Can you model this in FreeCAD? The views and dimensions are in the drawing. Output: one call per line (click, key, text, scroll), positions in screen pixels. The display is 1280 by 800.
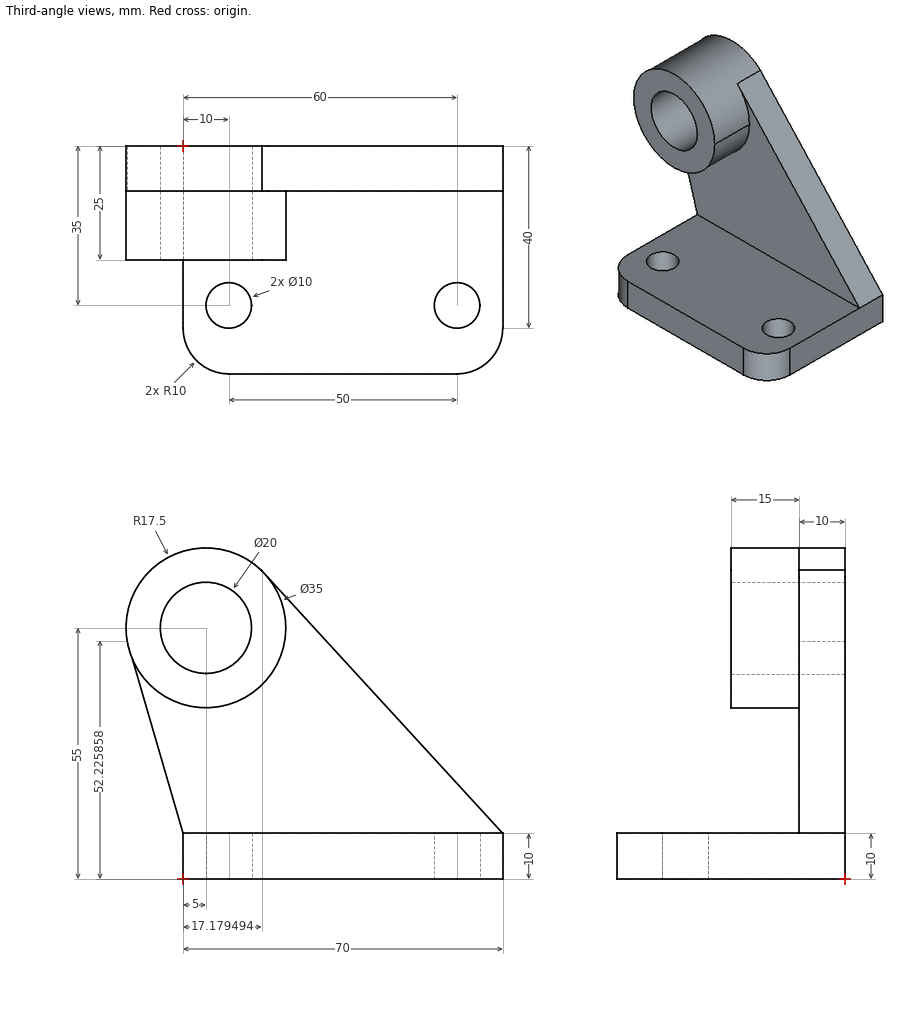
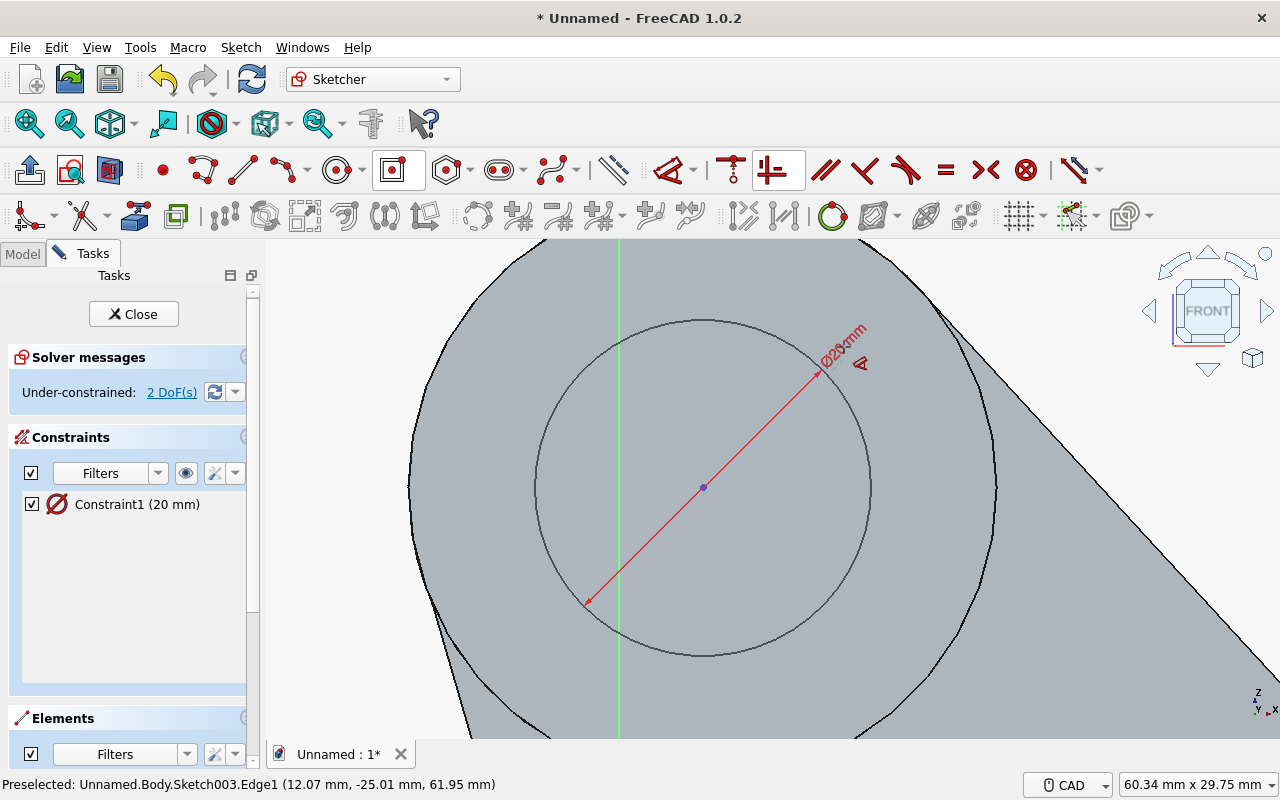
click(703, 488)
click(661, 454)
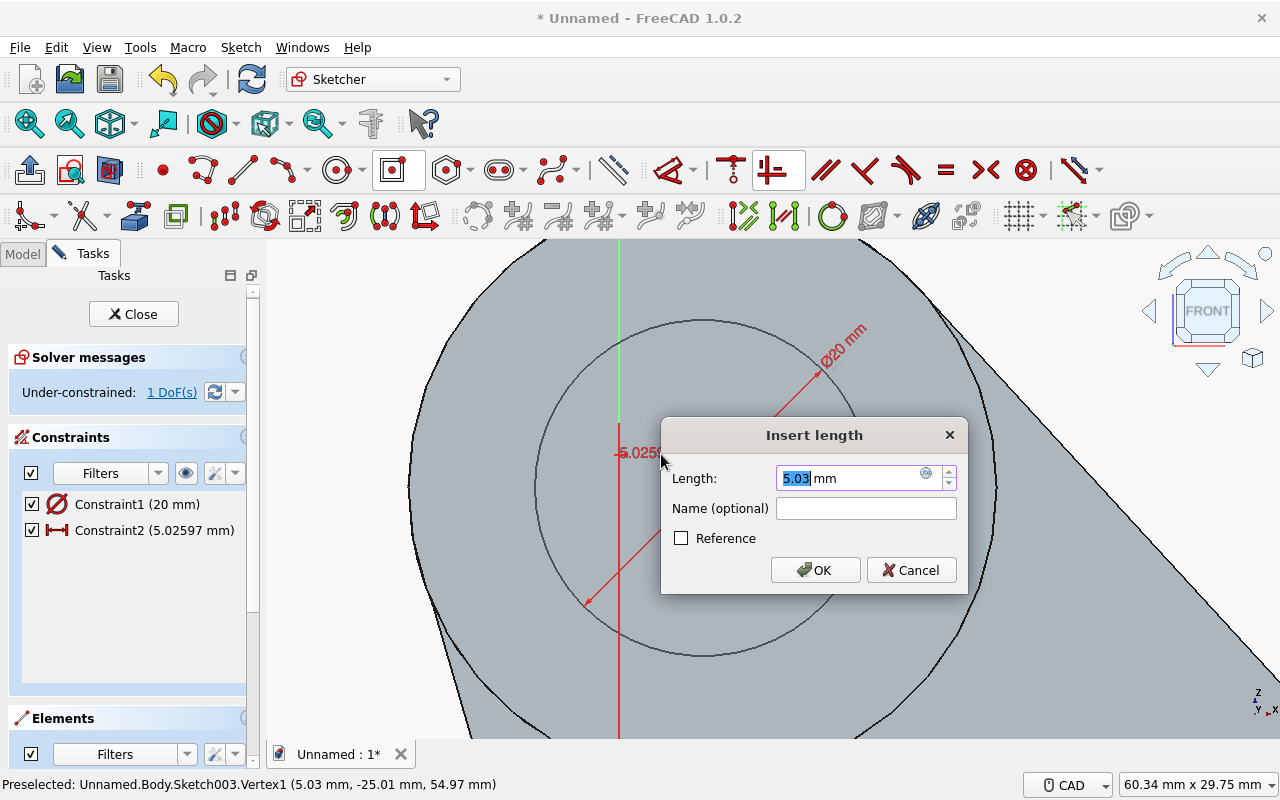
text(5)
key(Return)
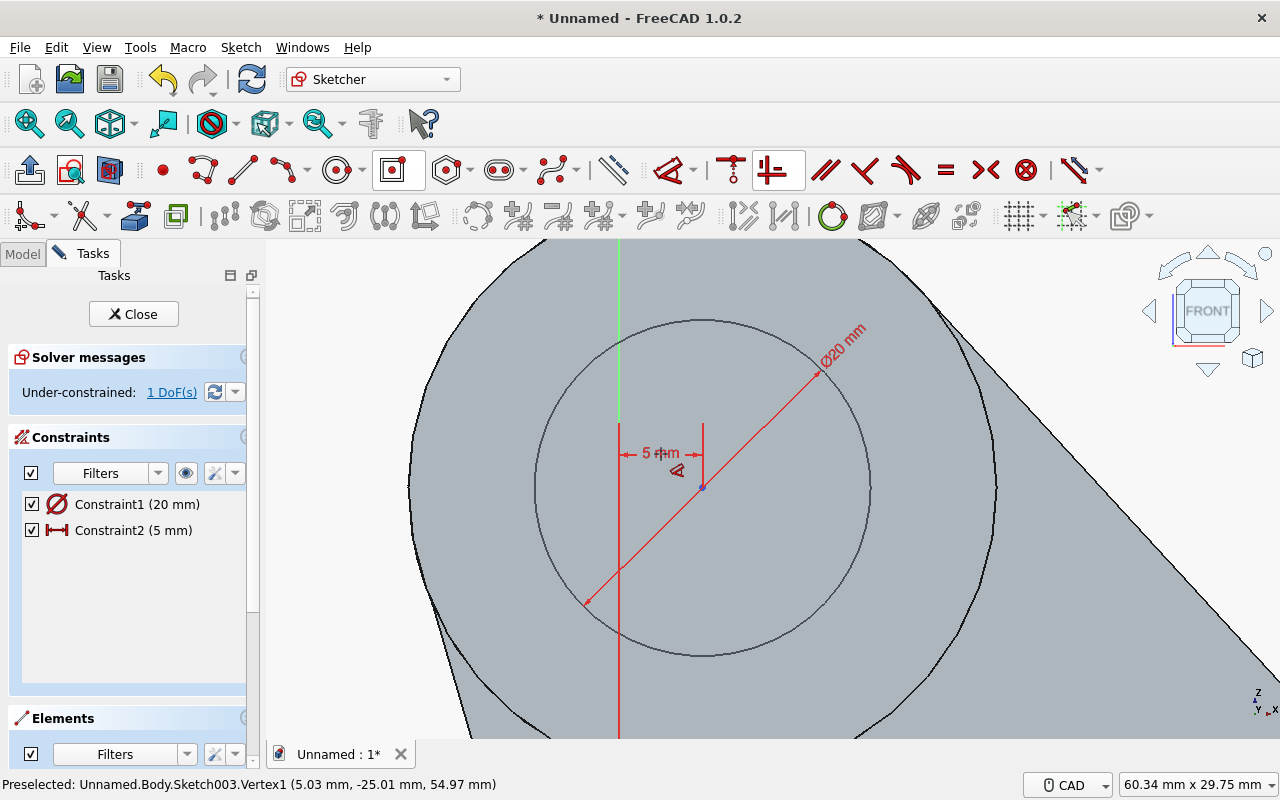
click(703, 488)
click(585, 548)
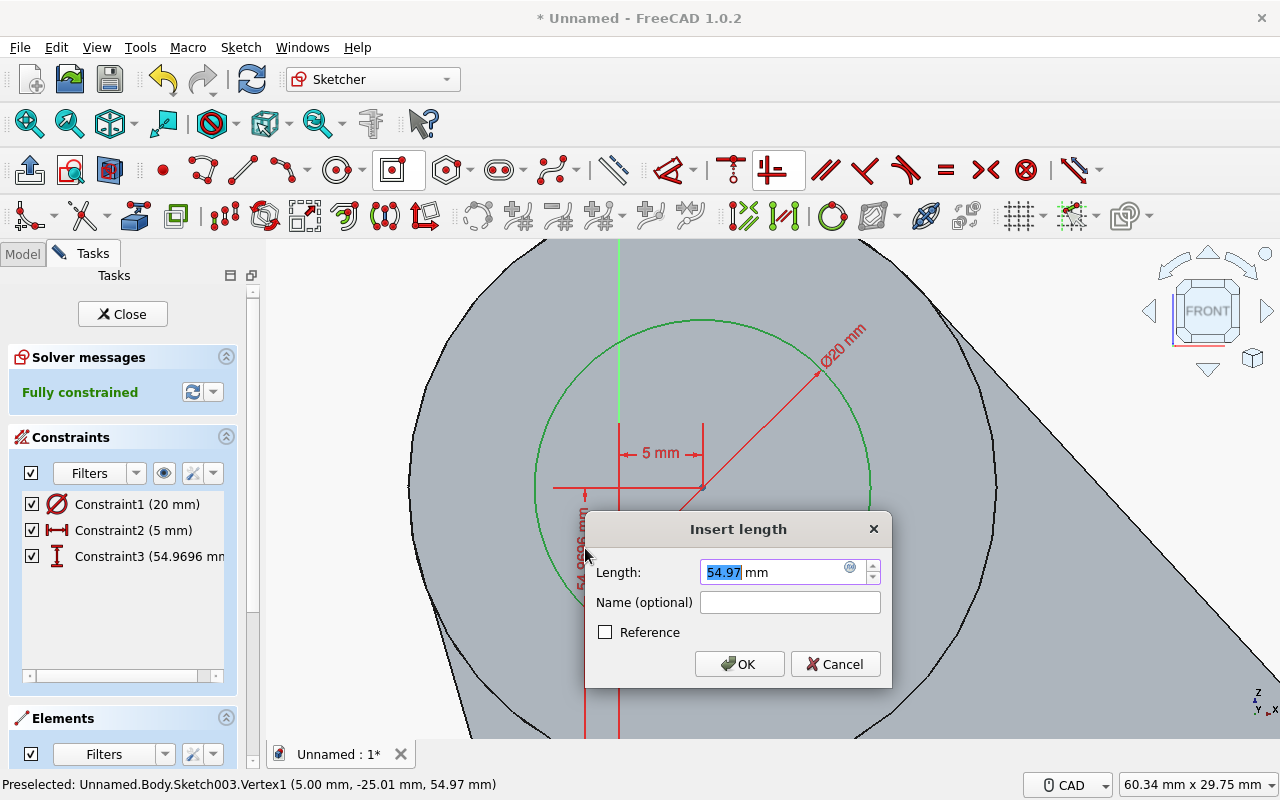
text(55)
key(Return)
key(Escape)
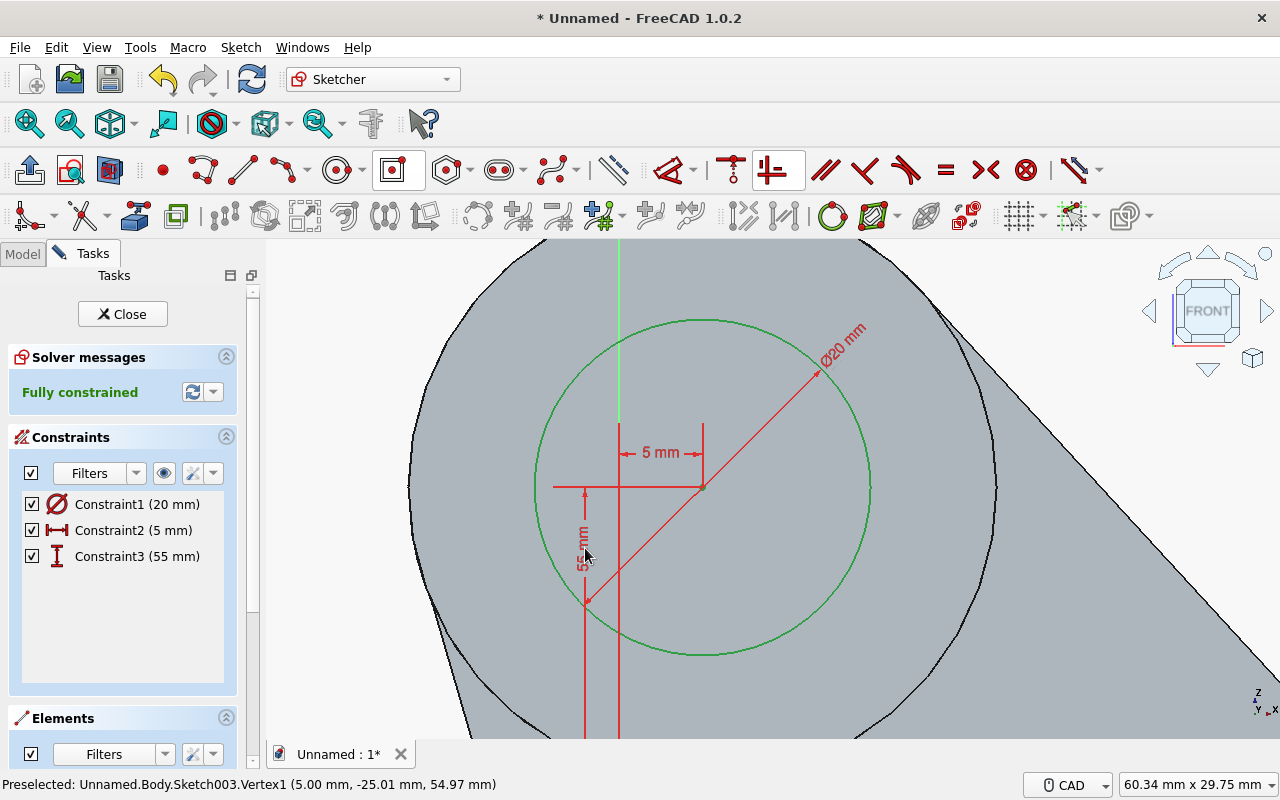
click(123, 314)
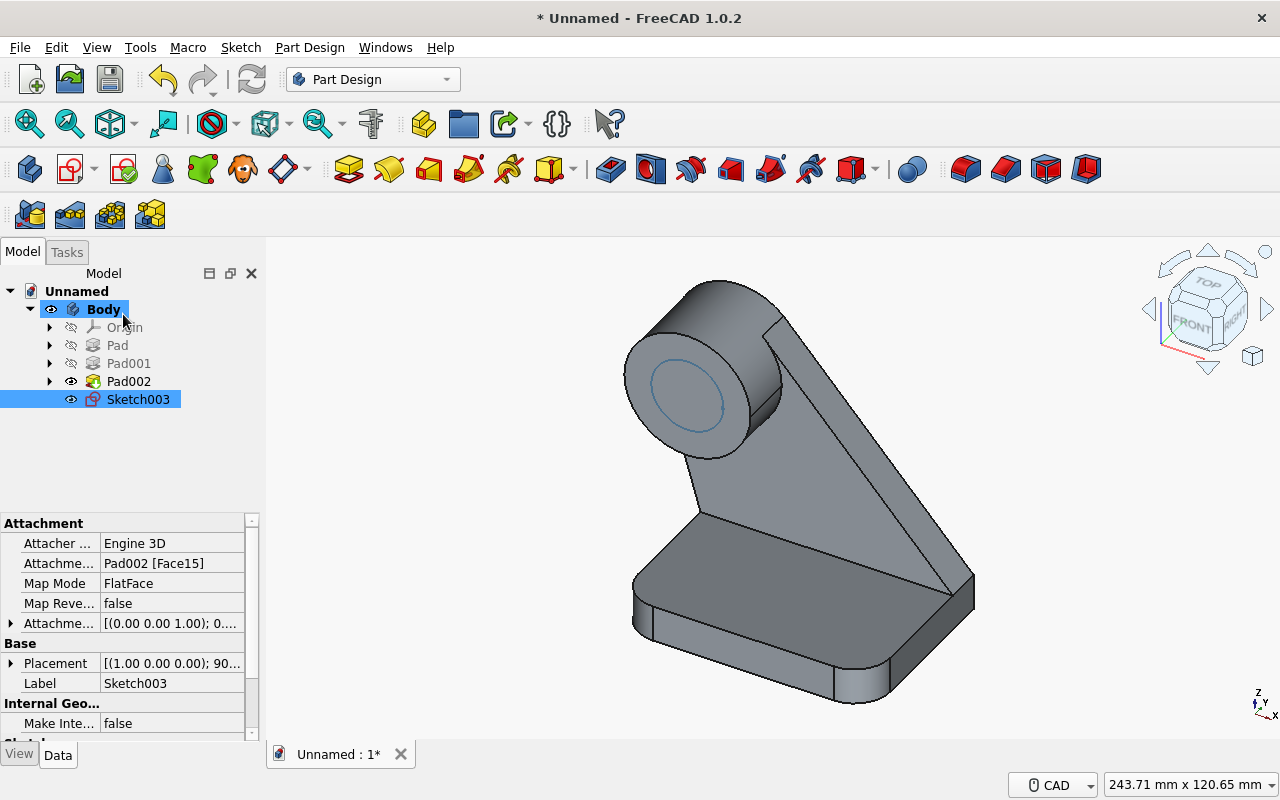
click(612, 170)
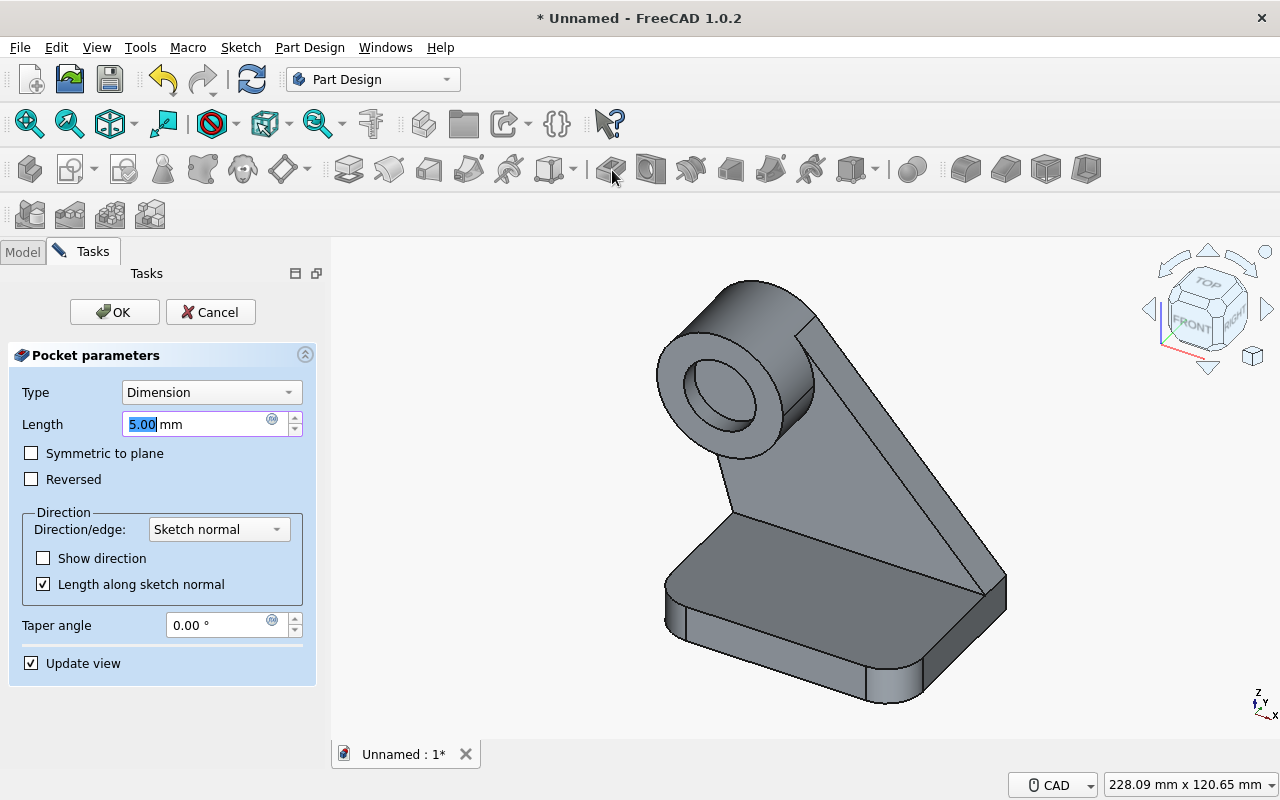
text(25)
key(Tab)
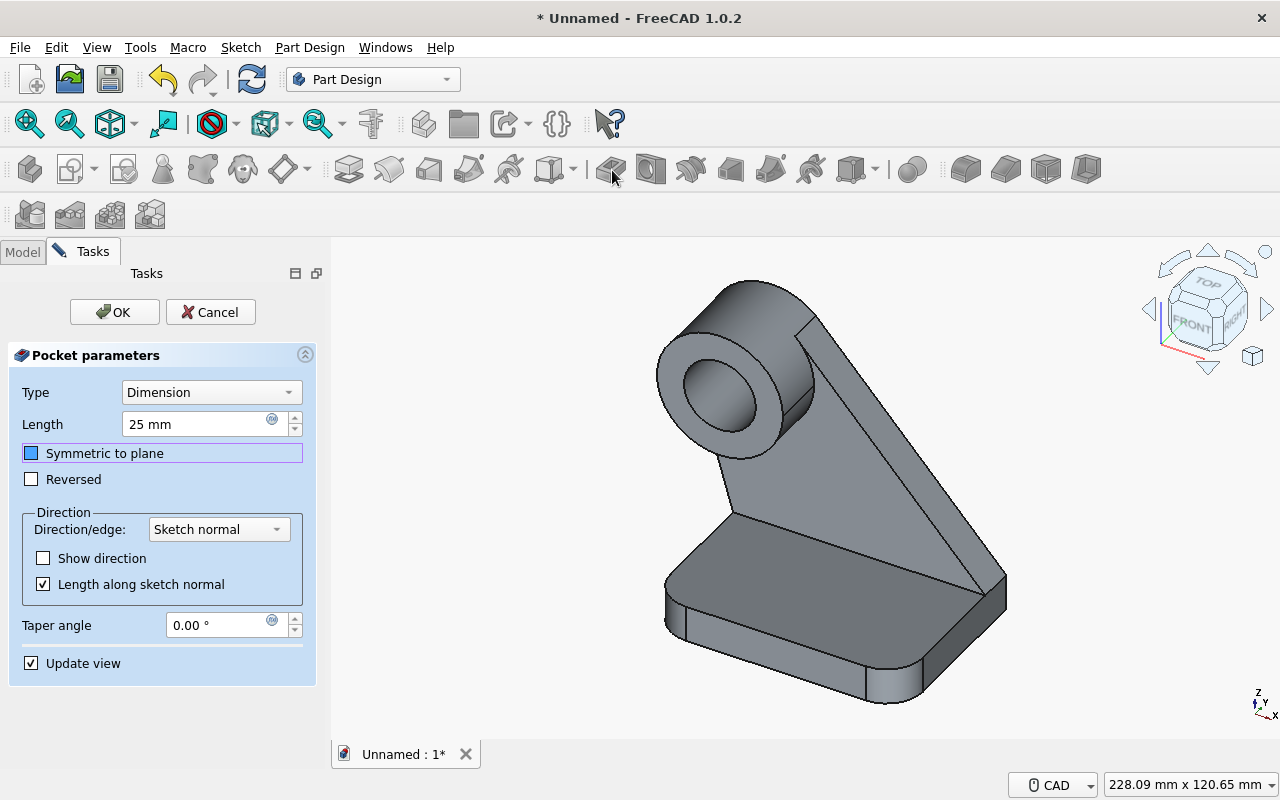
click(115, 312)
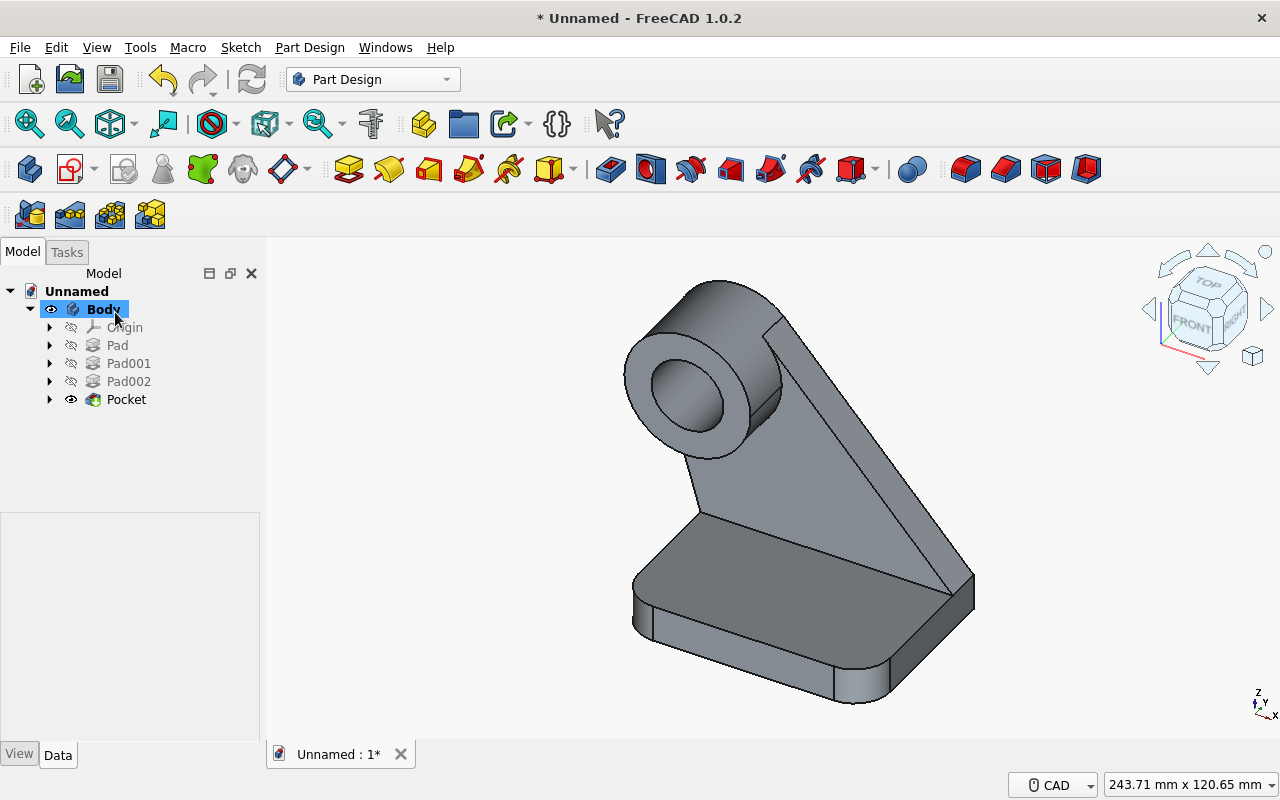
click(821, 606)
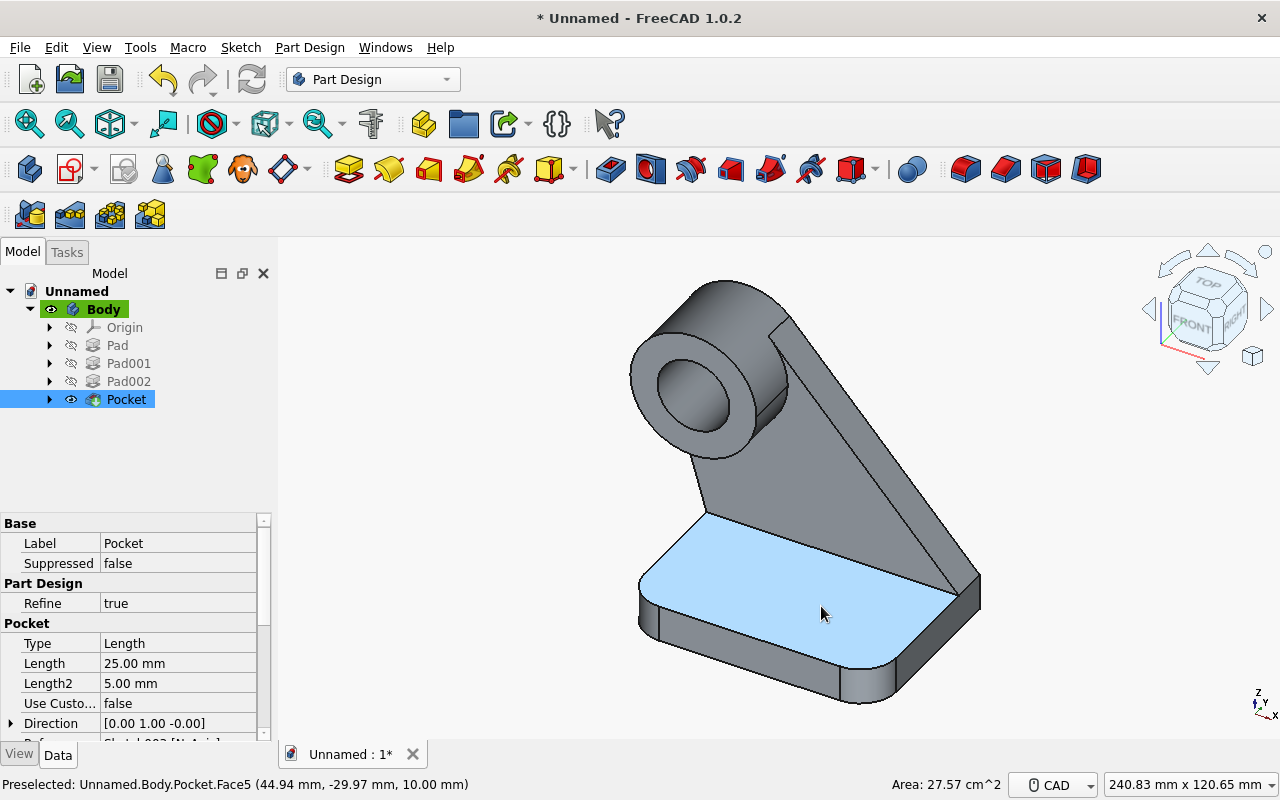
click(70, 170)